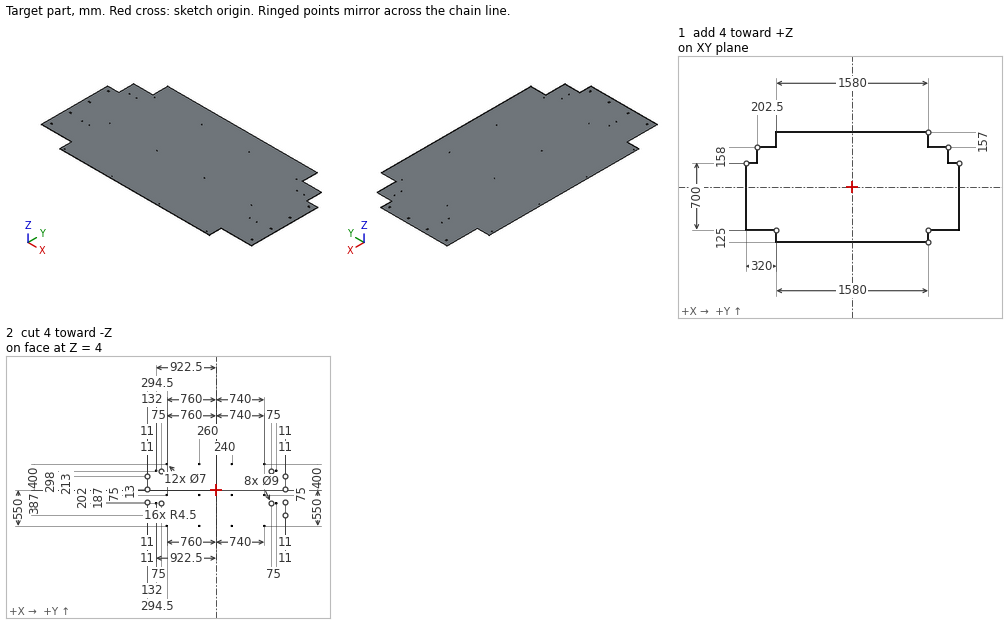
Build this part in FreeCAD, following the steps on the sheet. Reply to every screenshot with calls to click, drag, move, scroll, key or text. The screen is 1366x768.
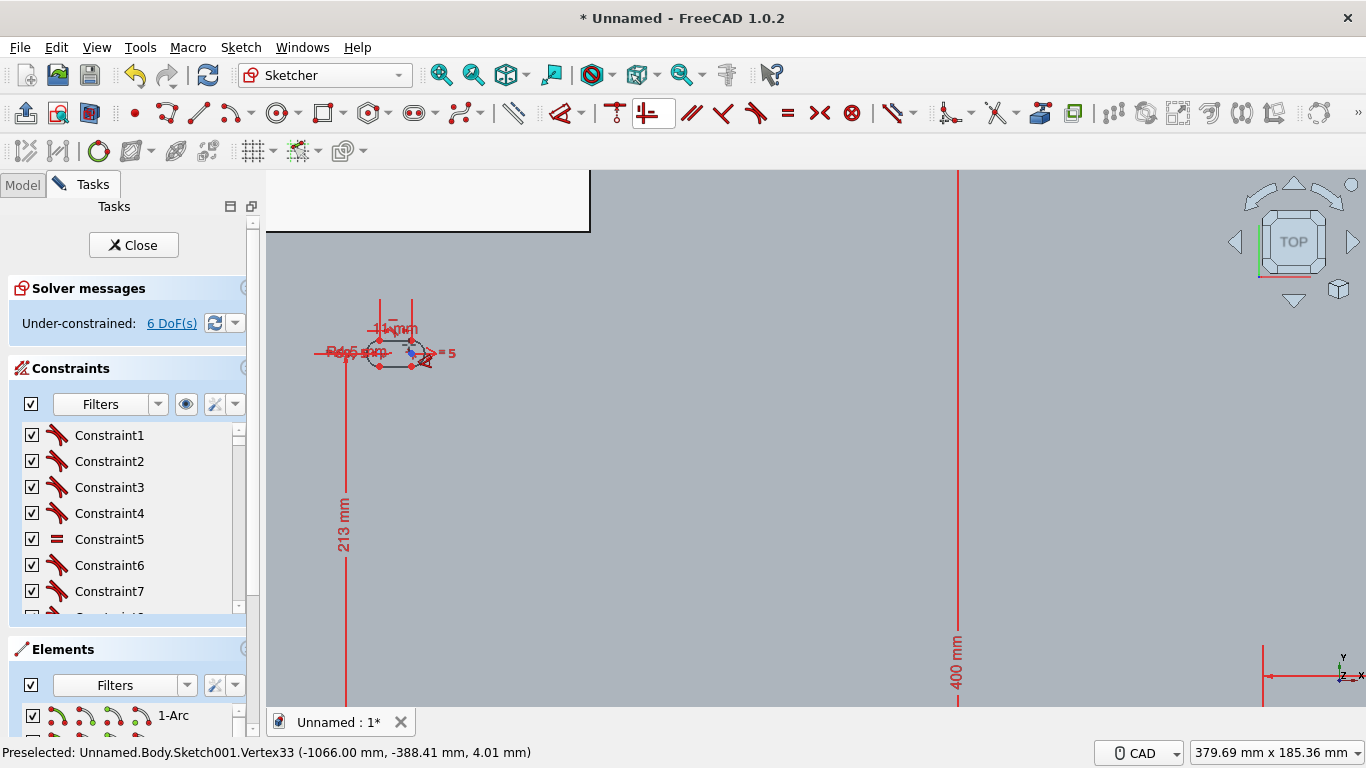
click(412, 341)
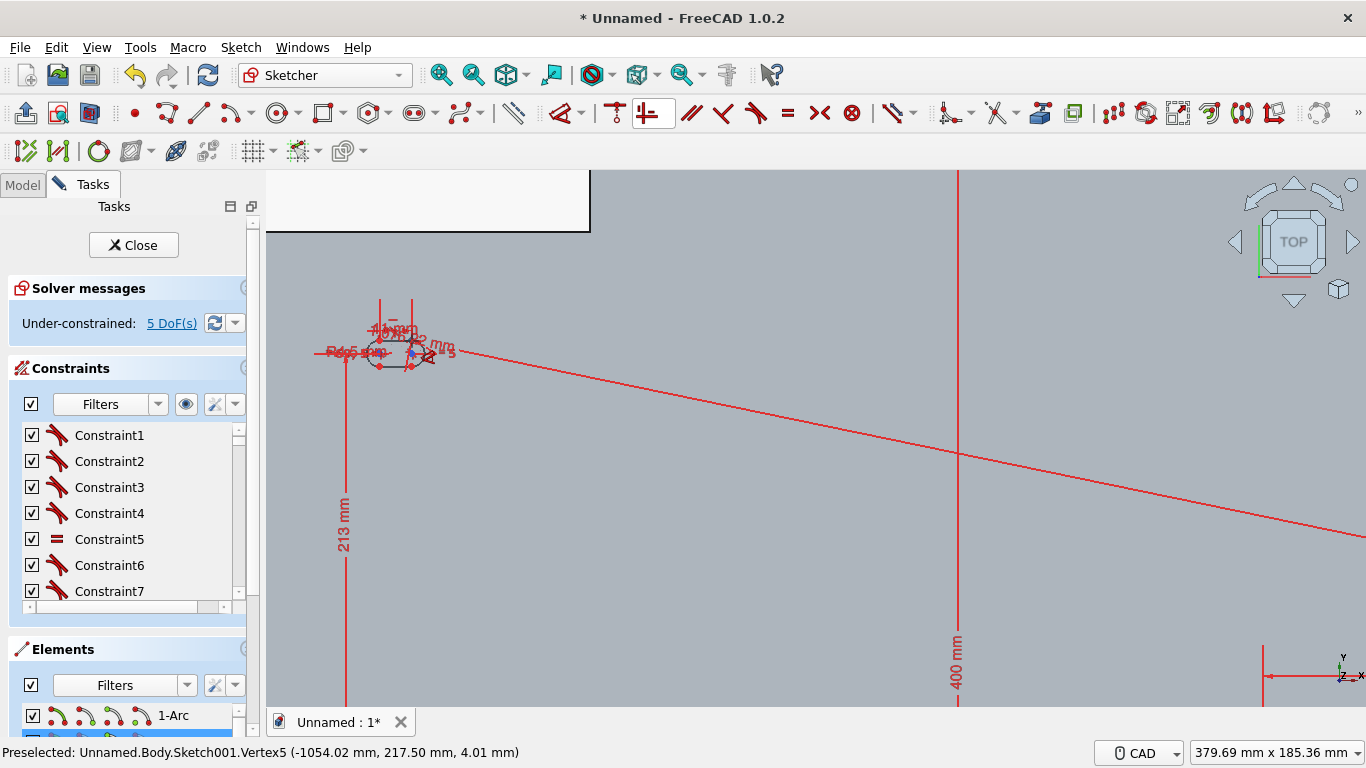
scroll(409, 345, down, 11)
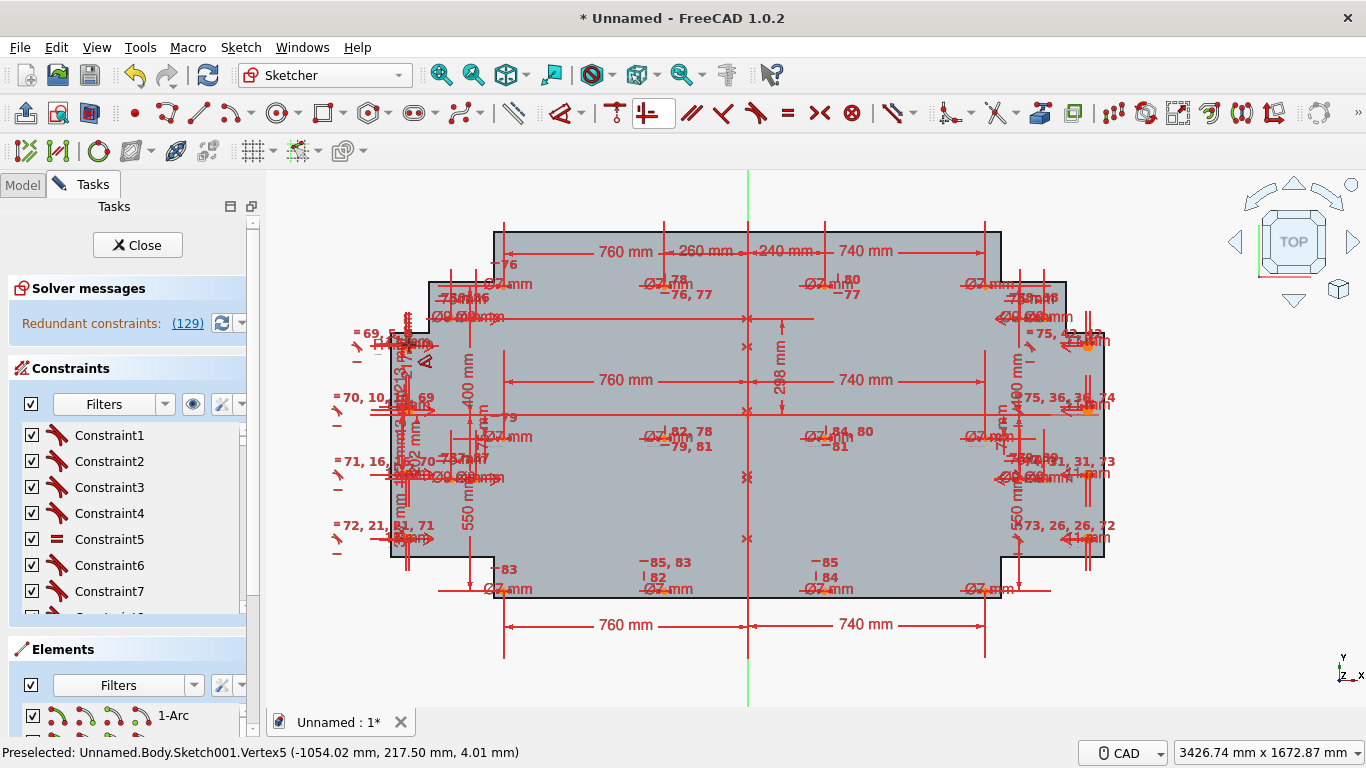
click(451, 319)
click(430, 261)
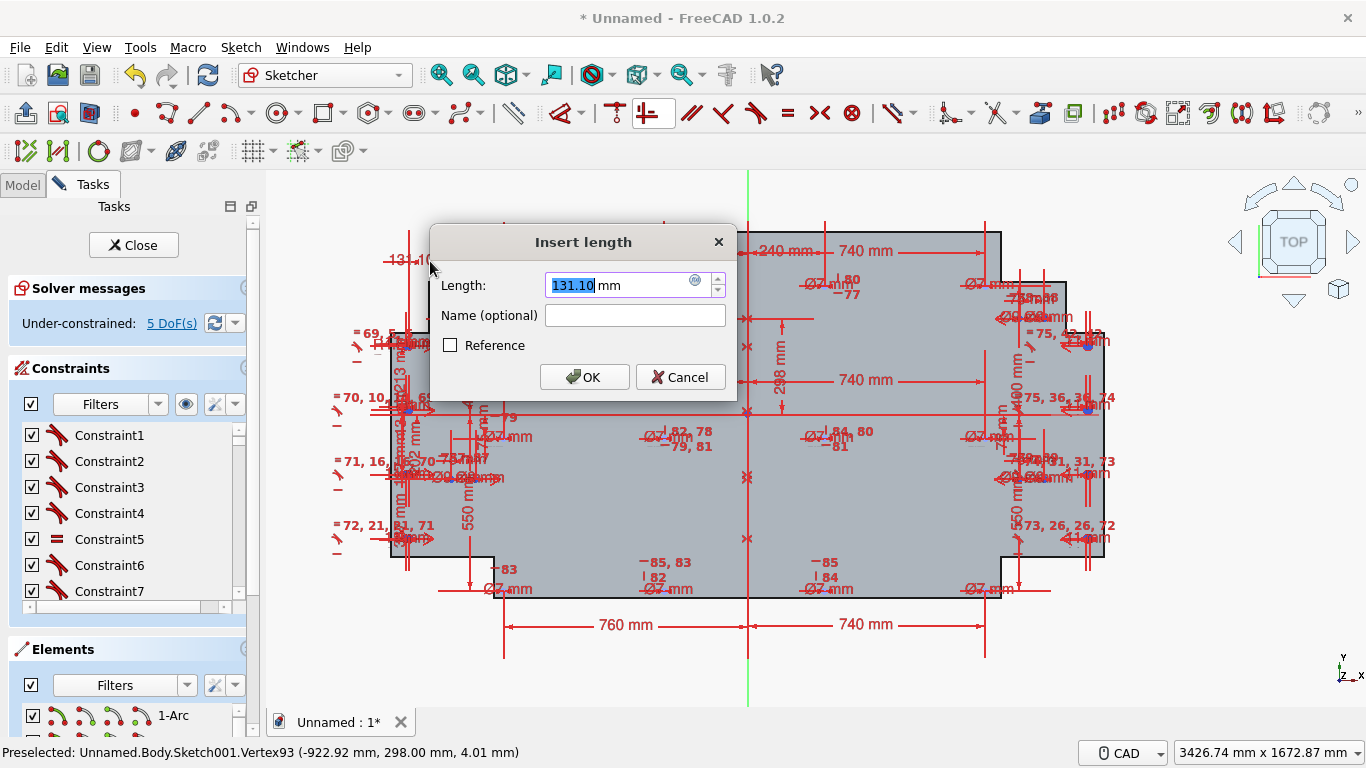
text(132)
key(Return)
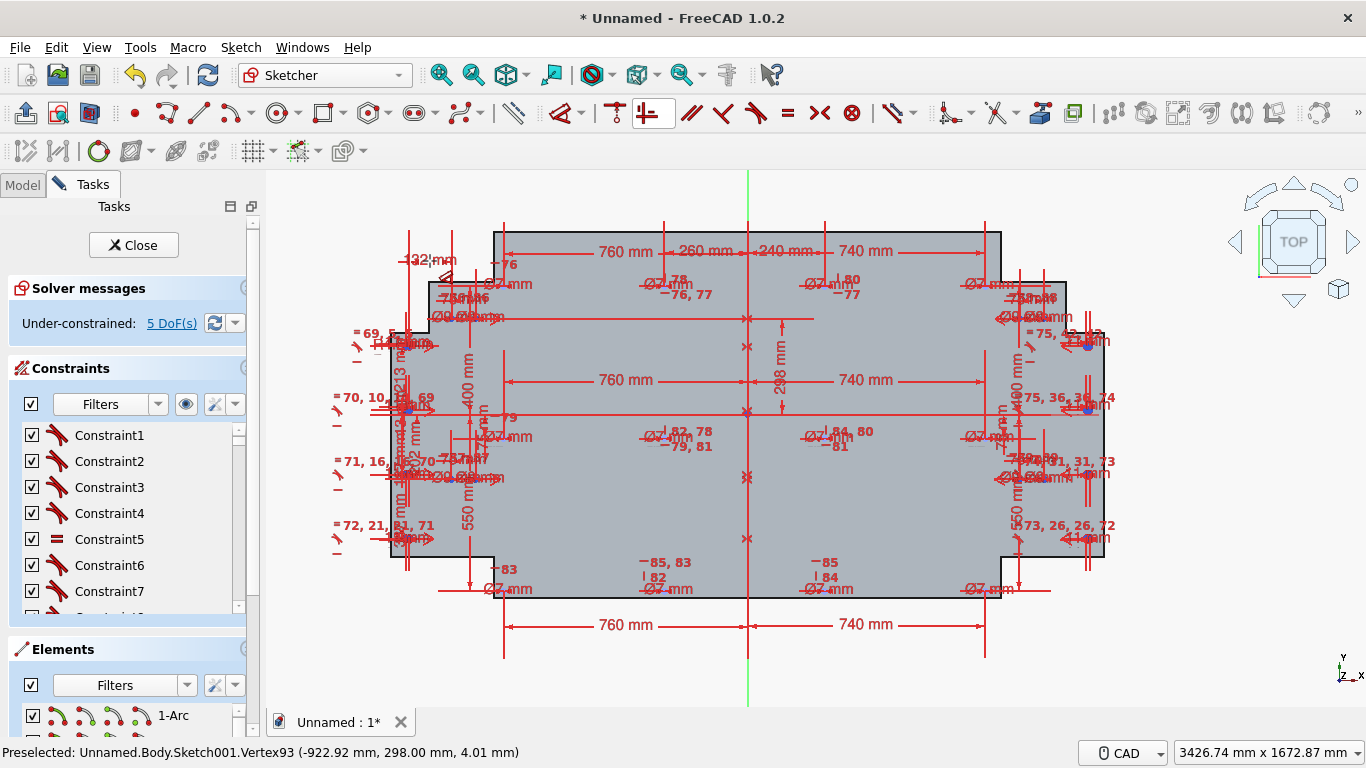
scroll(409, 476, up, 11)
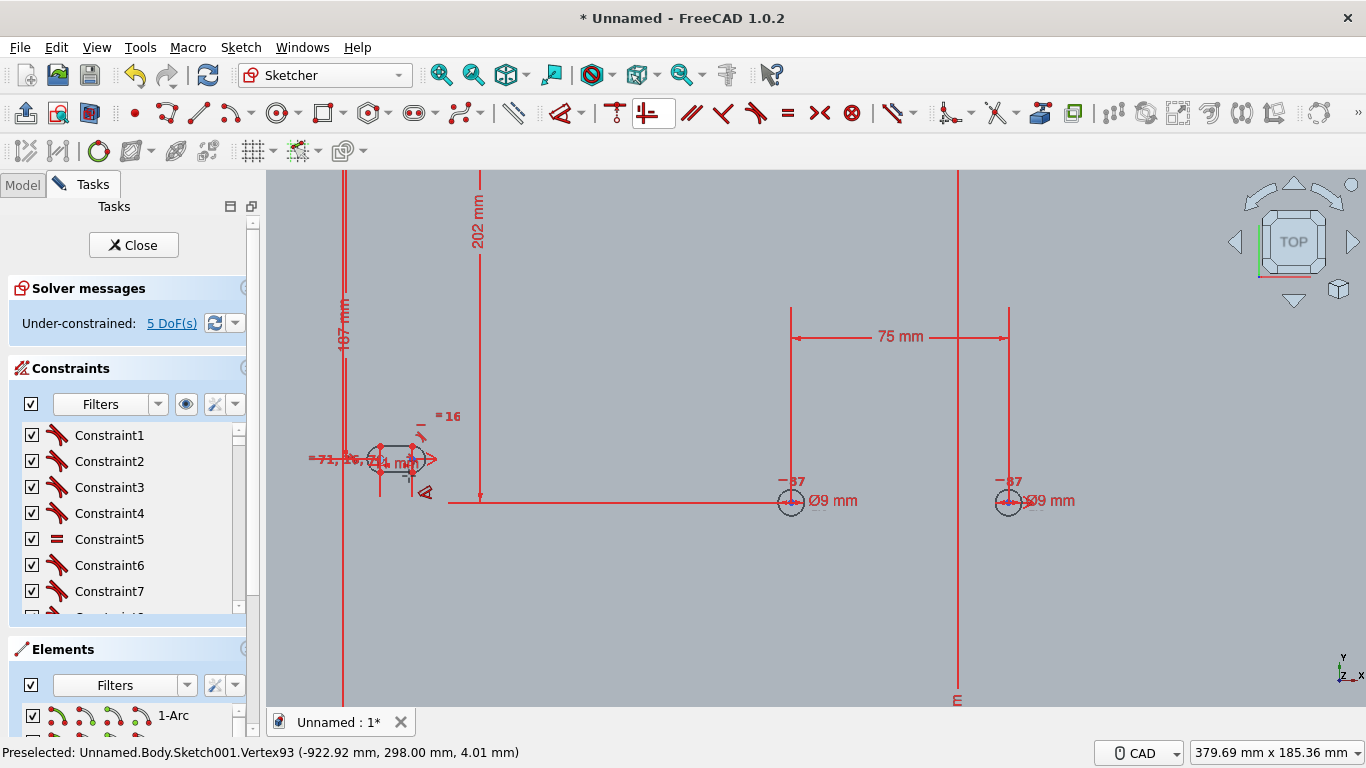
click(412, 472)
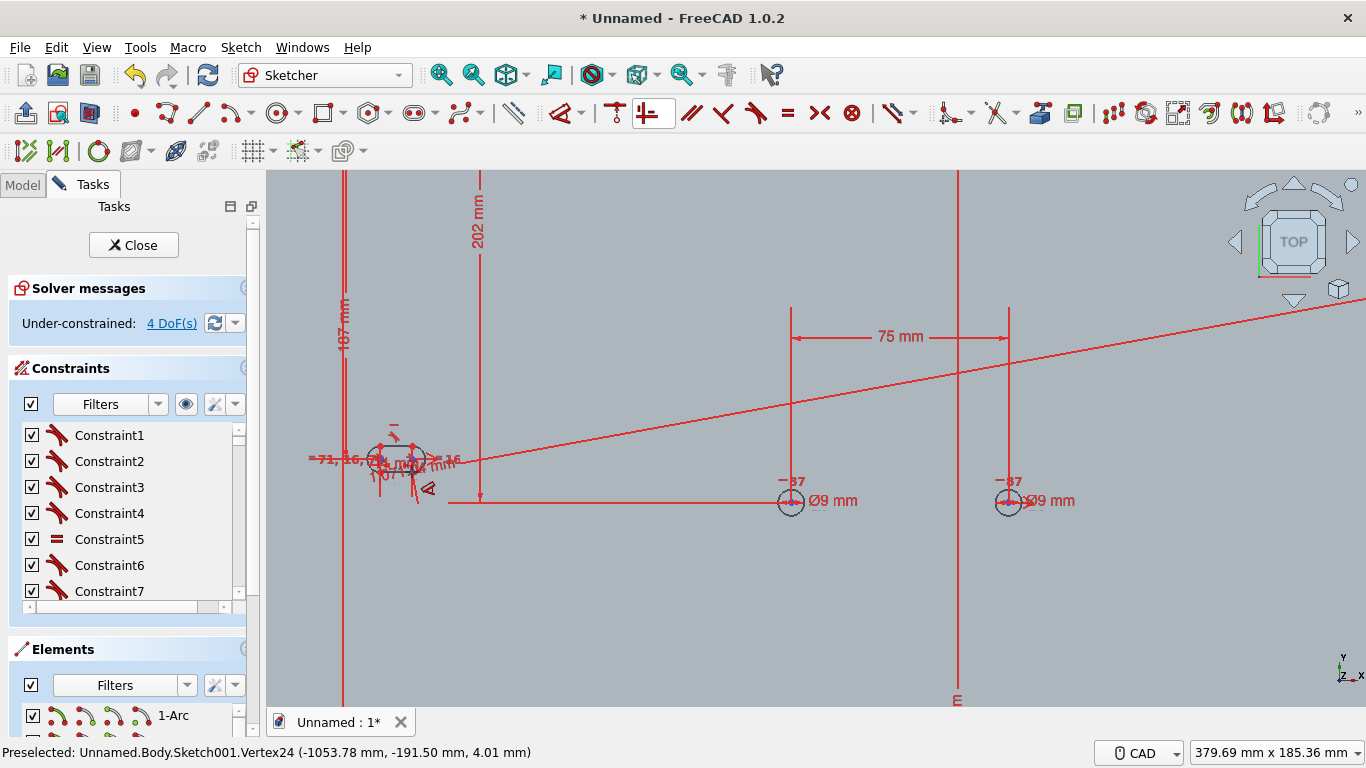
scroll(409, 476, down, 11)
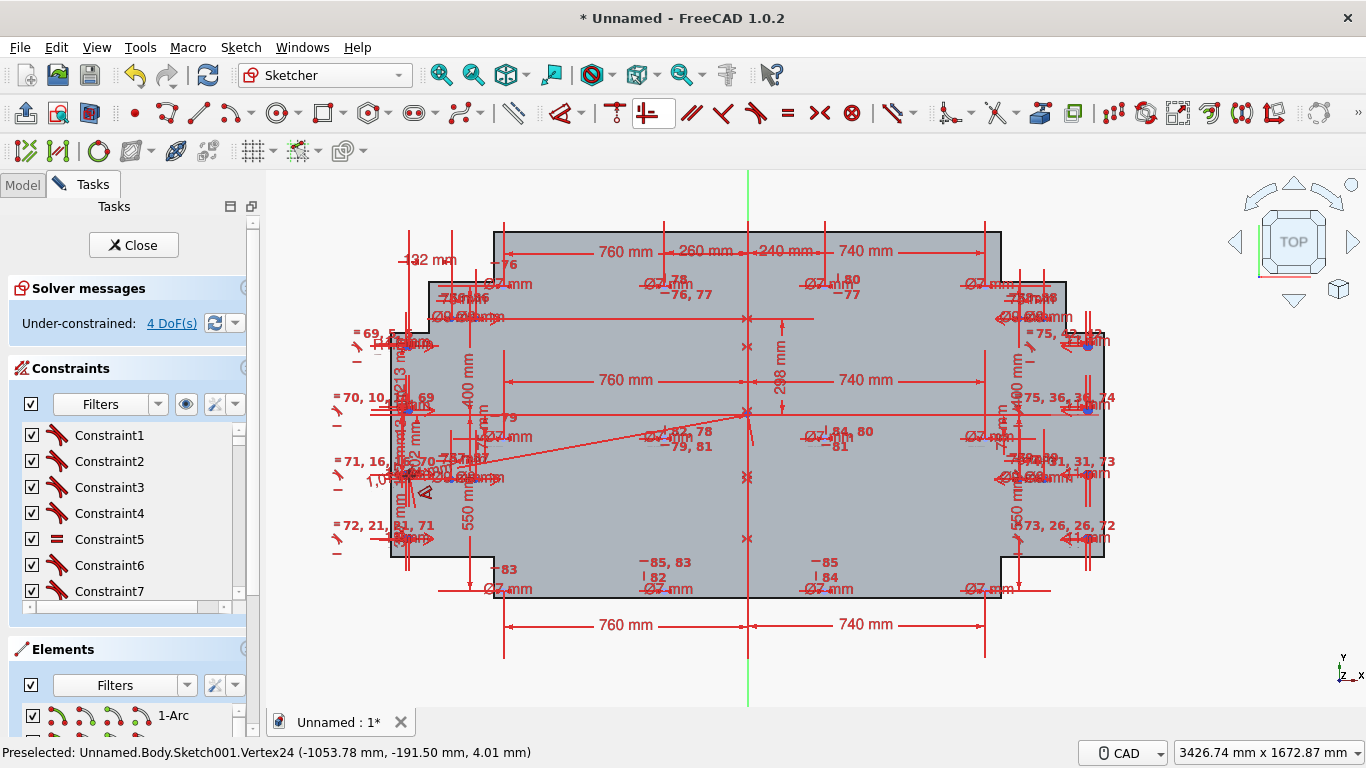
click(451, 479)
click(430, 561)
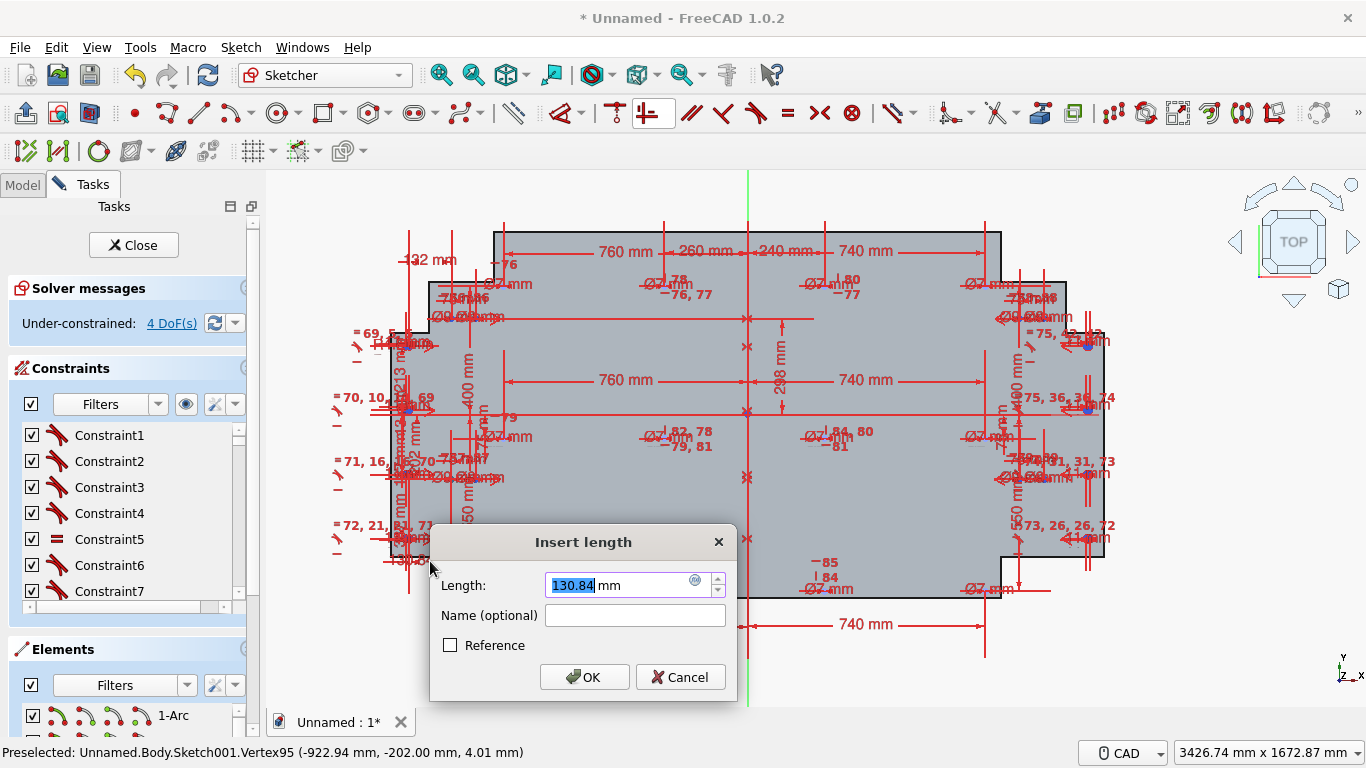
text(132)
key(Return)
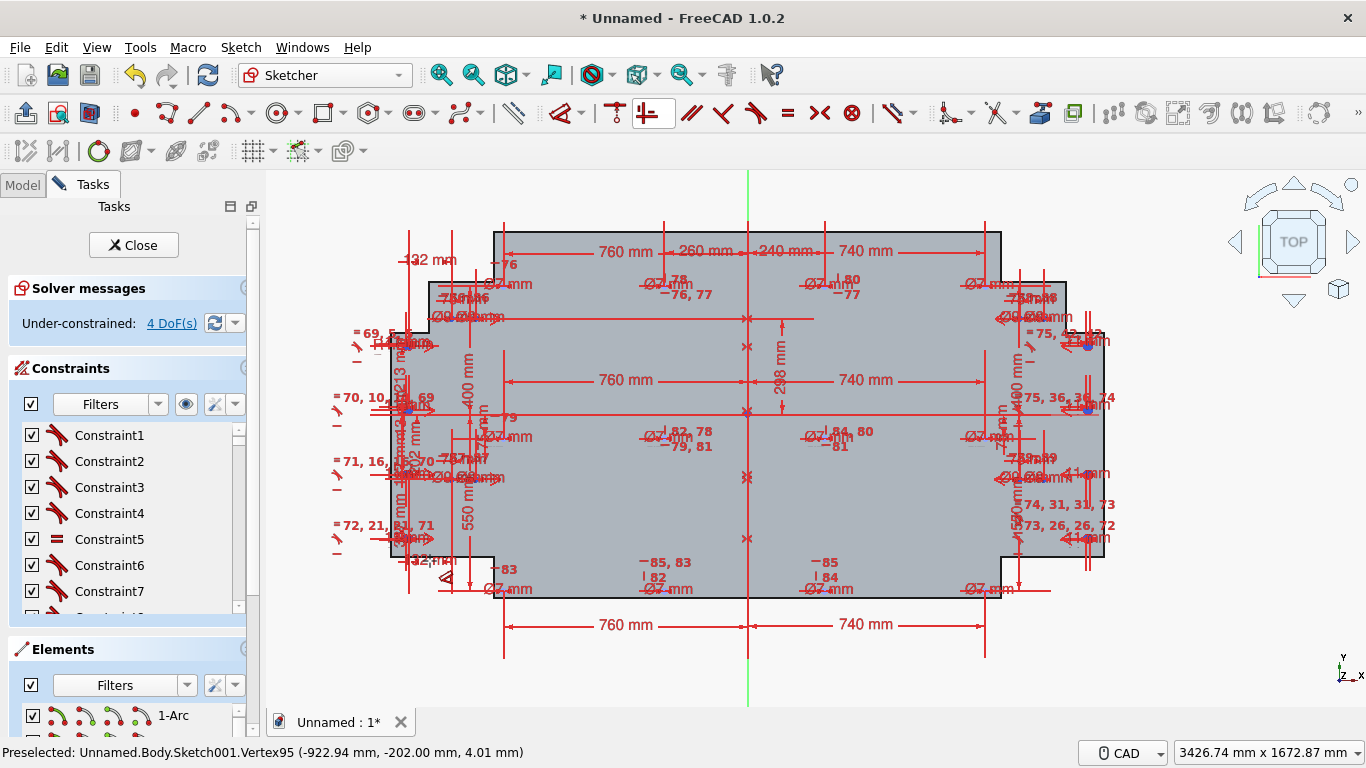
click(452, 319)
click(600, 285)